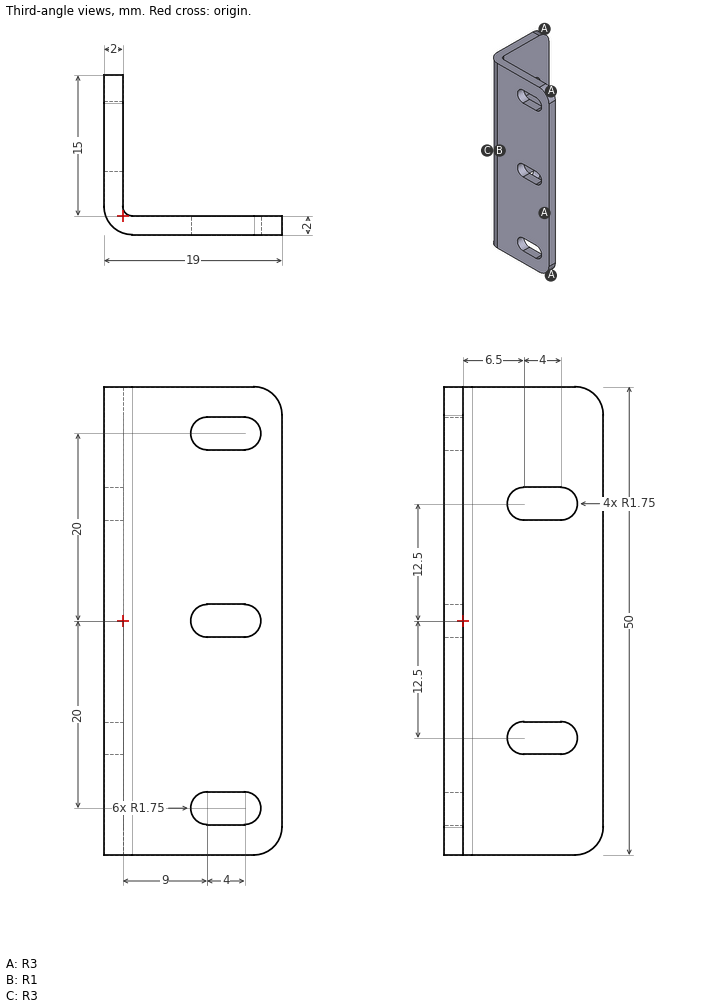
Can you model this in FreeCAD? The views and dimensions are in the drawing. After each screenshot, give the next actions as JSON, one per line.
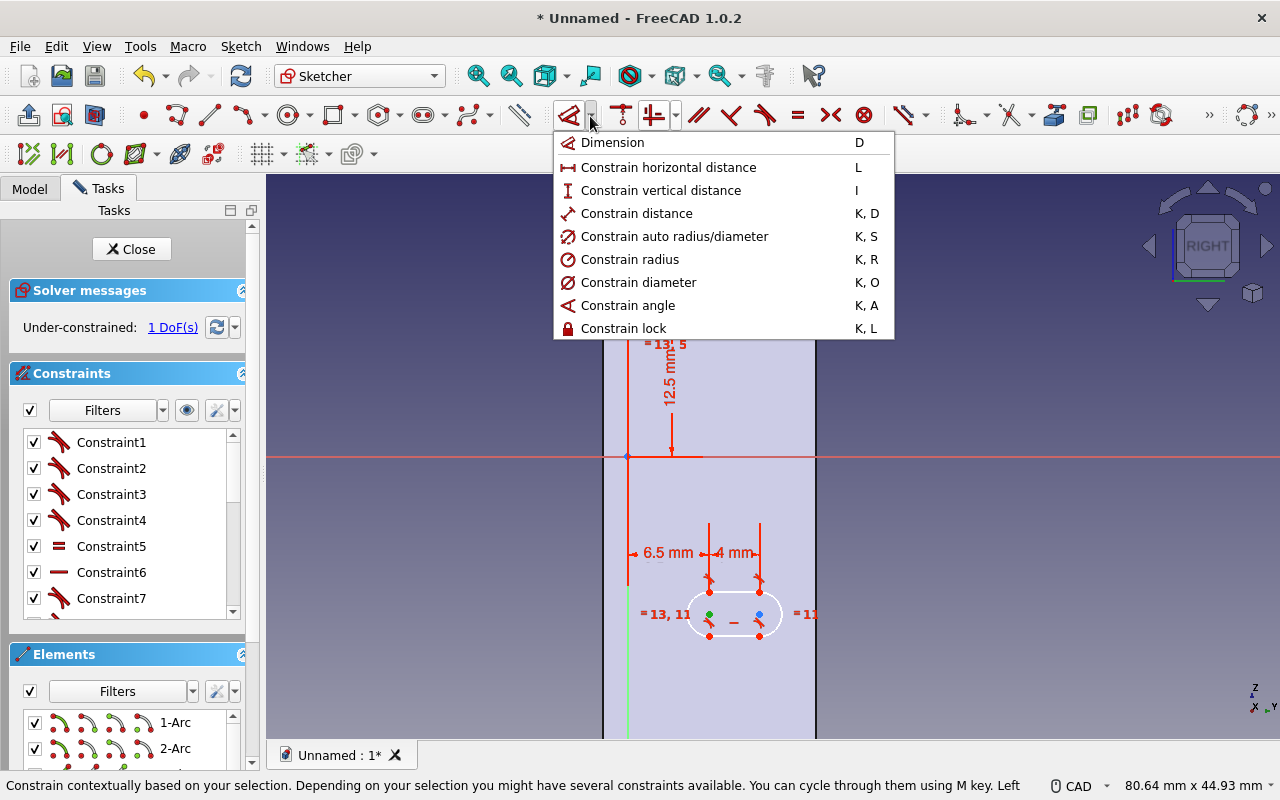
{"action": "left_click", "coordinate": [724, 190]}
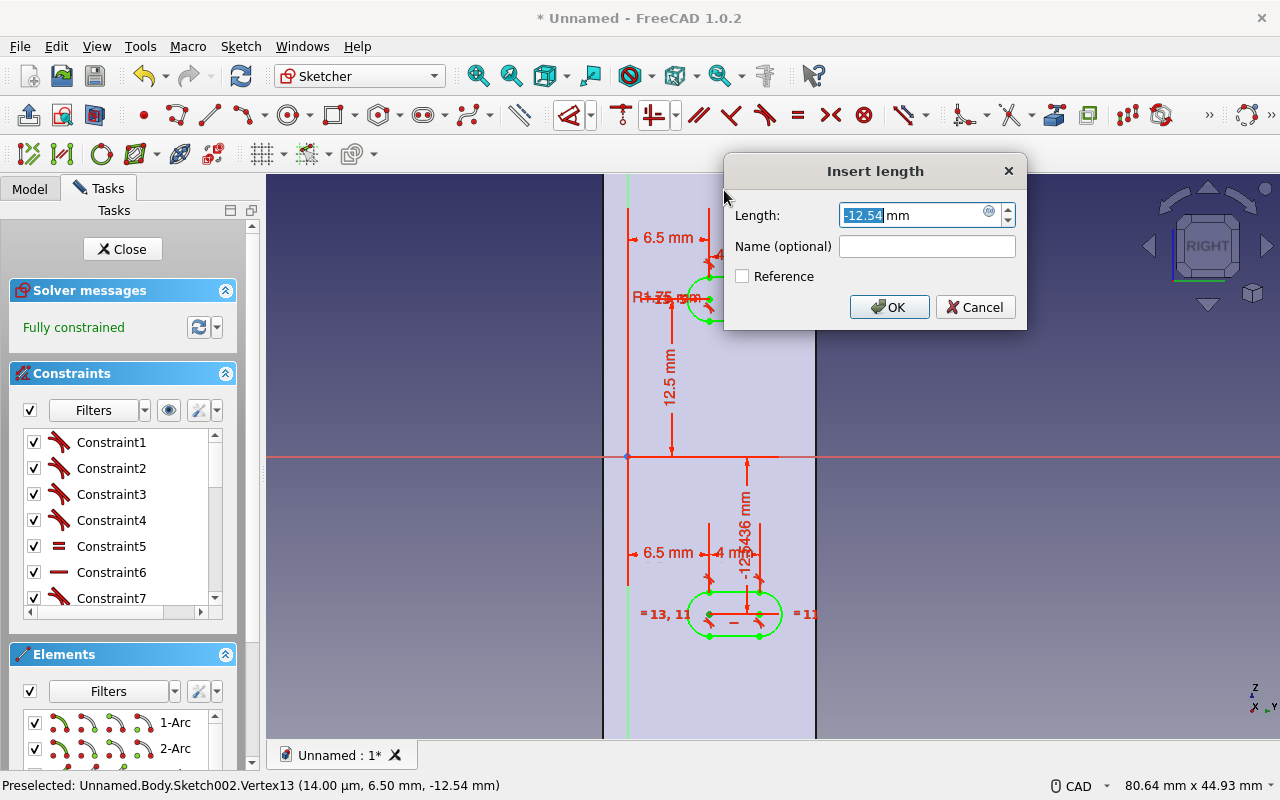
{"action": "type", "text": "-12.5"}
{"action": "key", "text": "Return"}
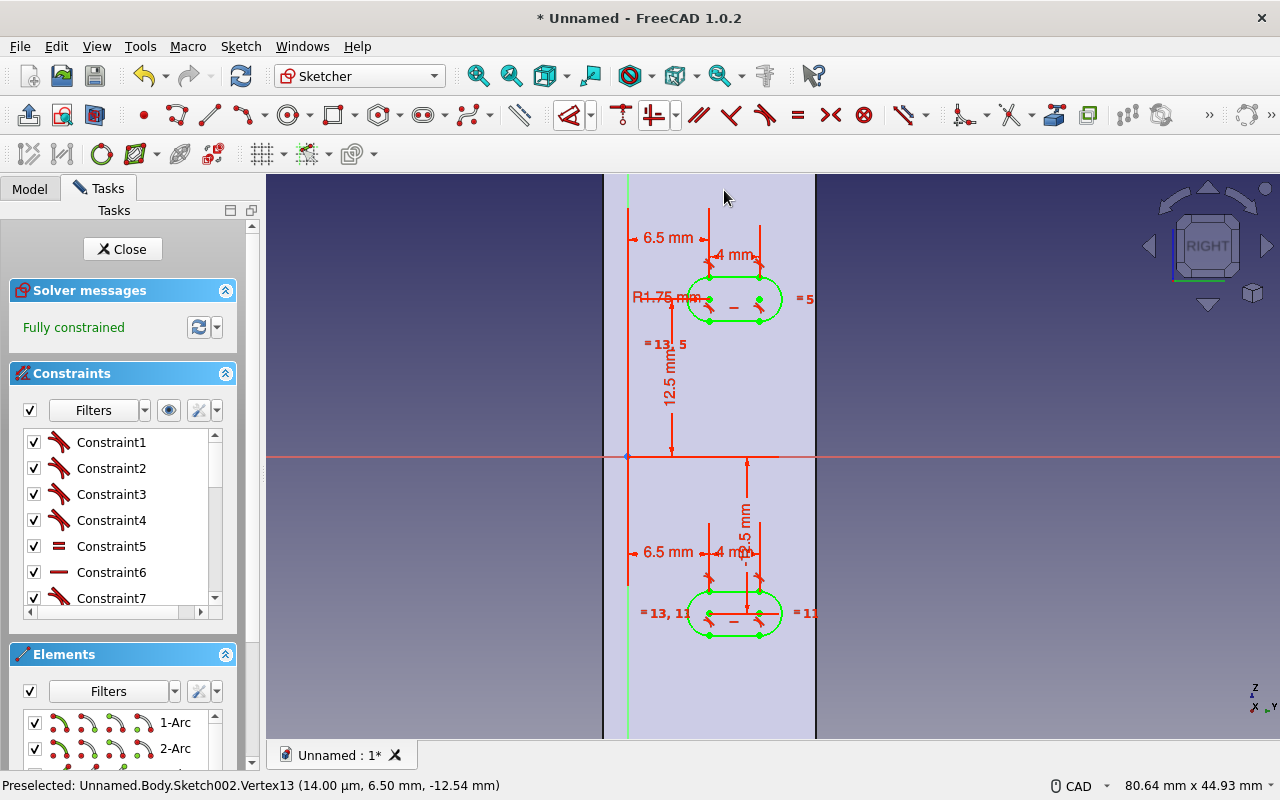
{"action": "left_click", "coordinate": [123, 249]}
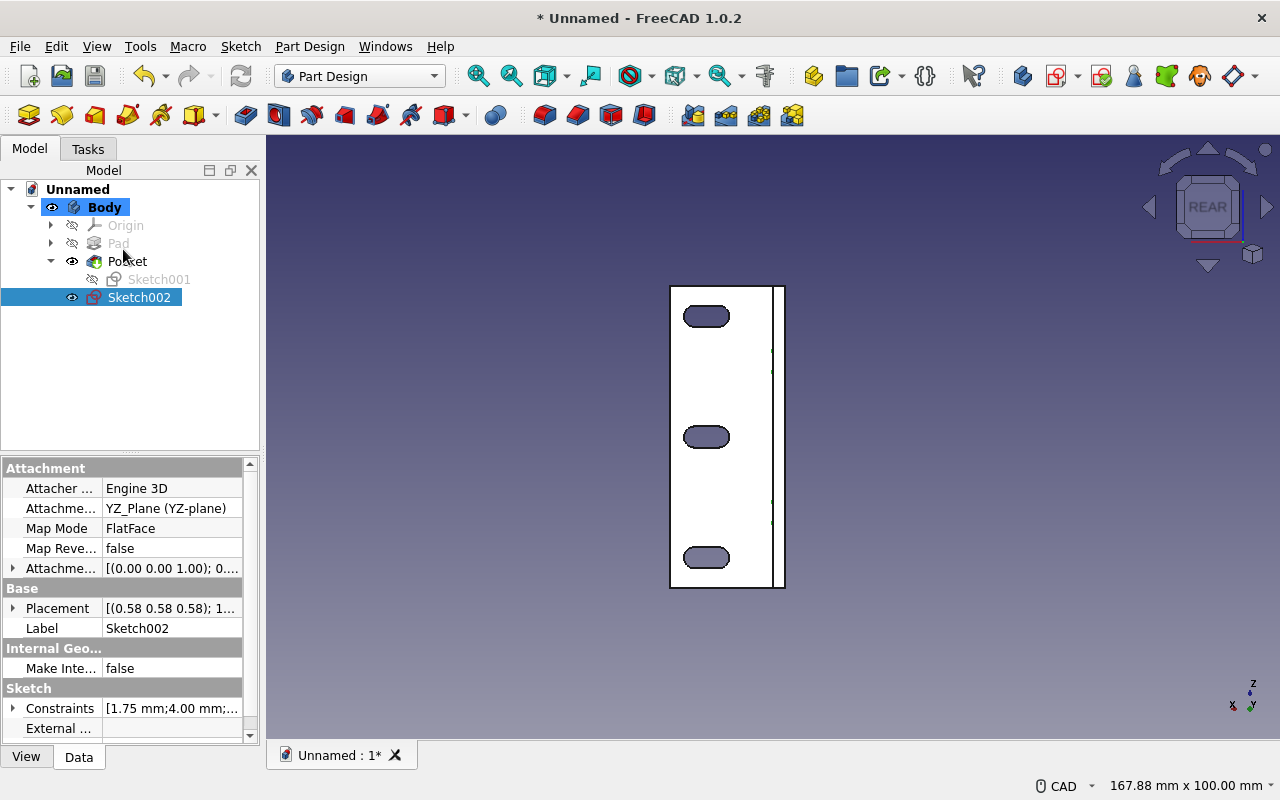
{"action": "left_click", "coordinate": [246, 116]}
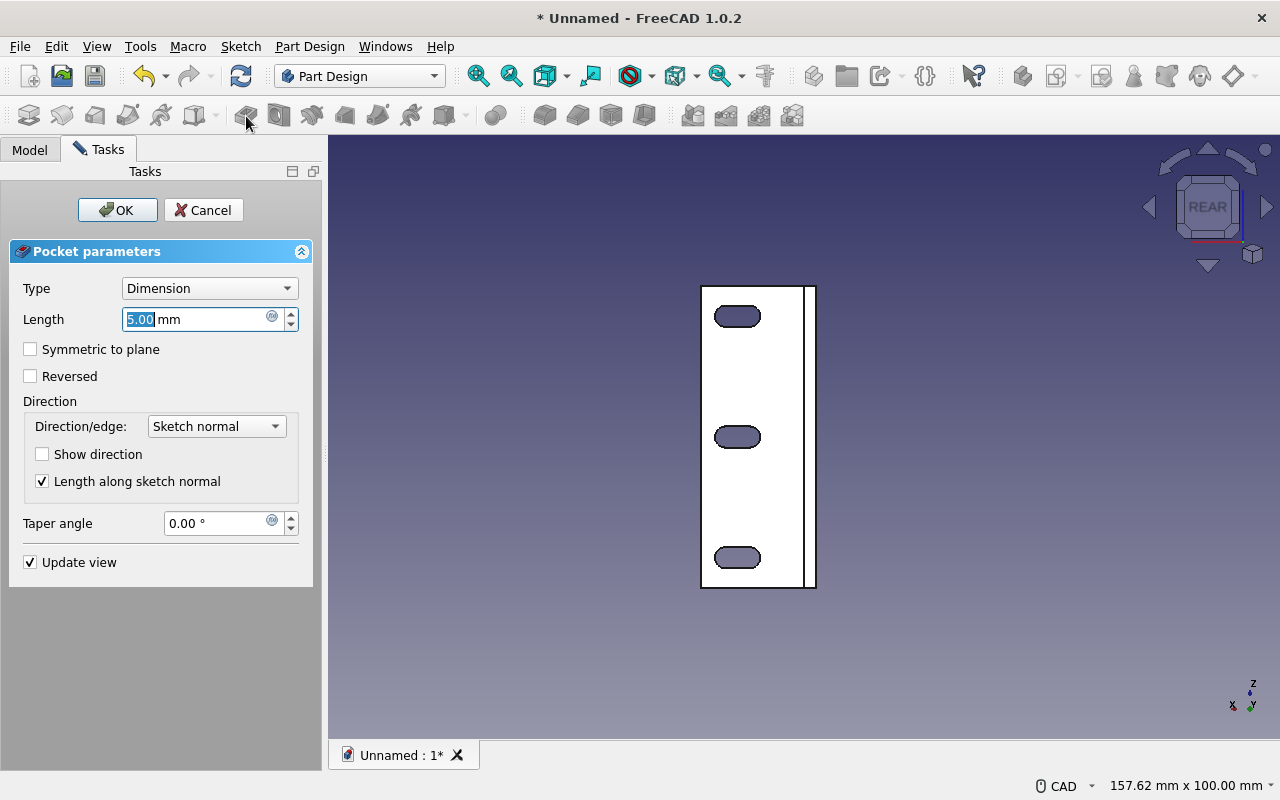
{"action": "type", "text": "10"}
{"action": "key", "text": "Tab"}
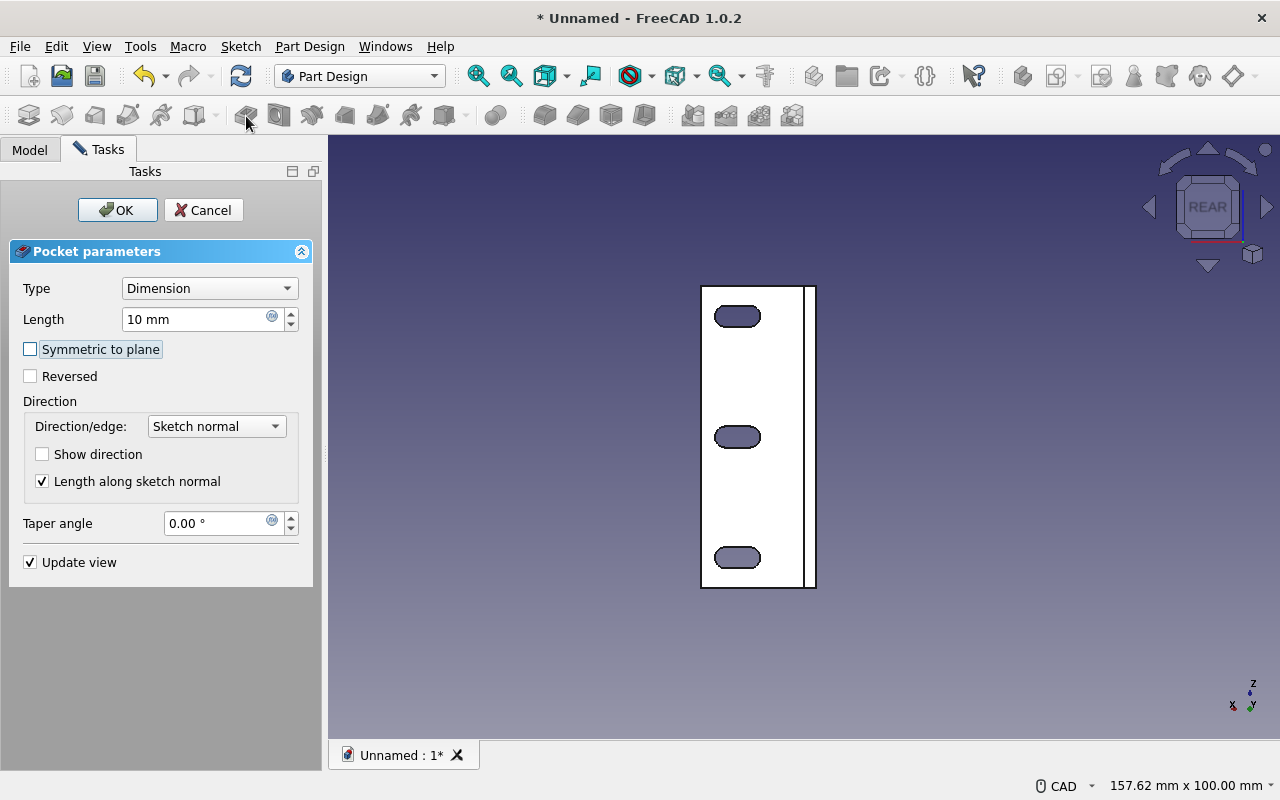
{"action": "left_click", "coordinate": [118, 210]}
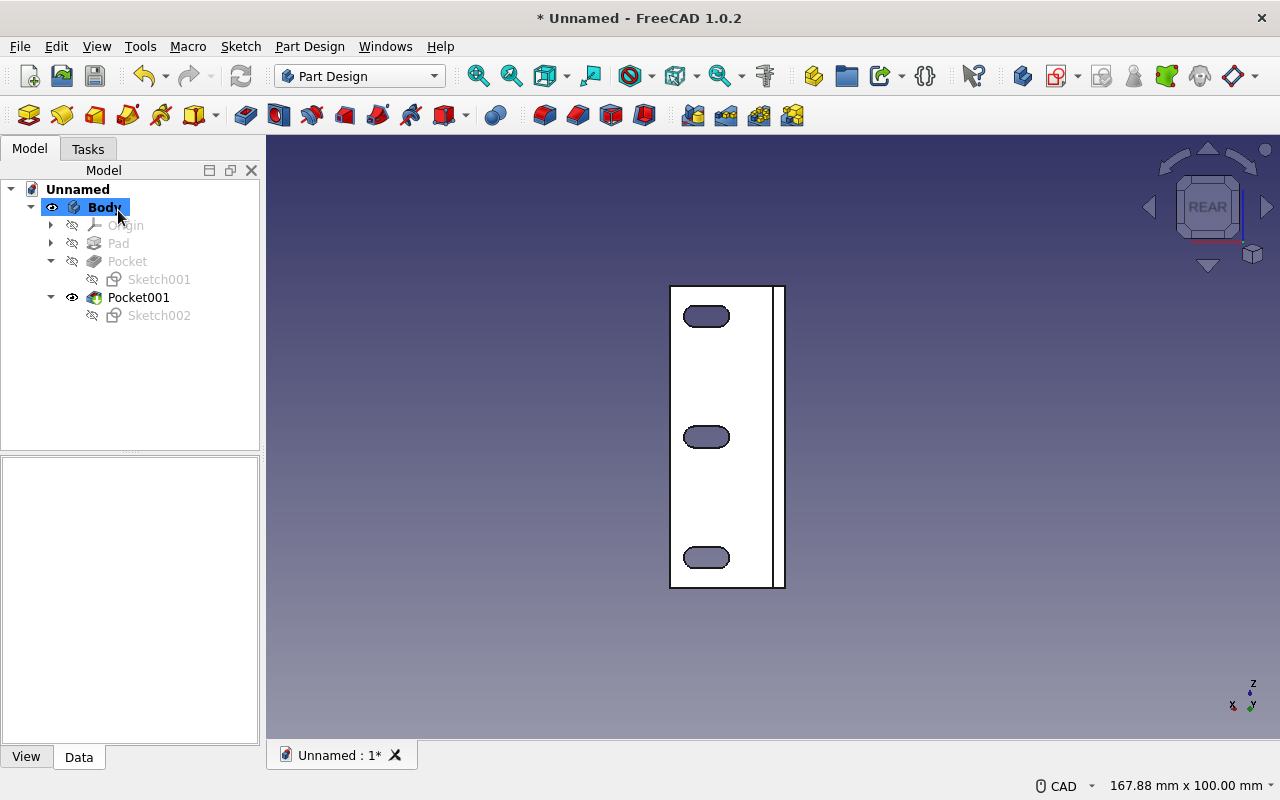
{"action": "left_click", "coordinate": [779, 285]}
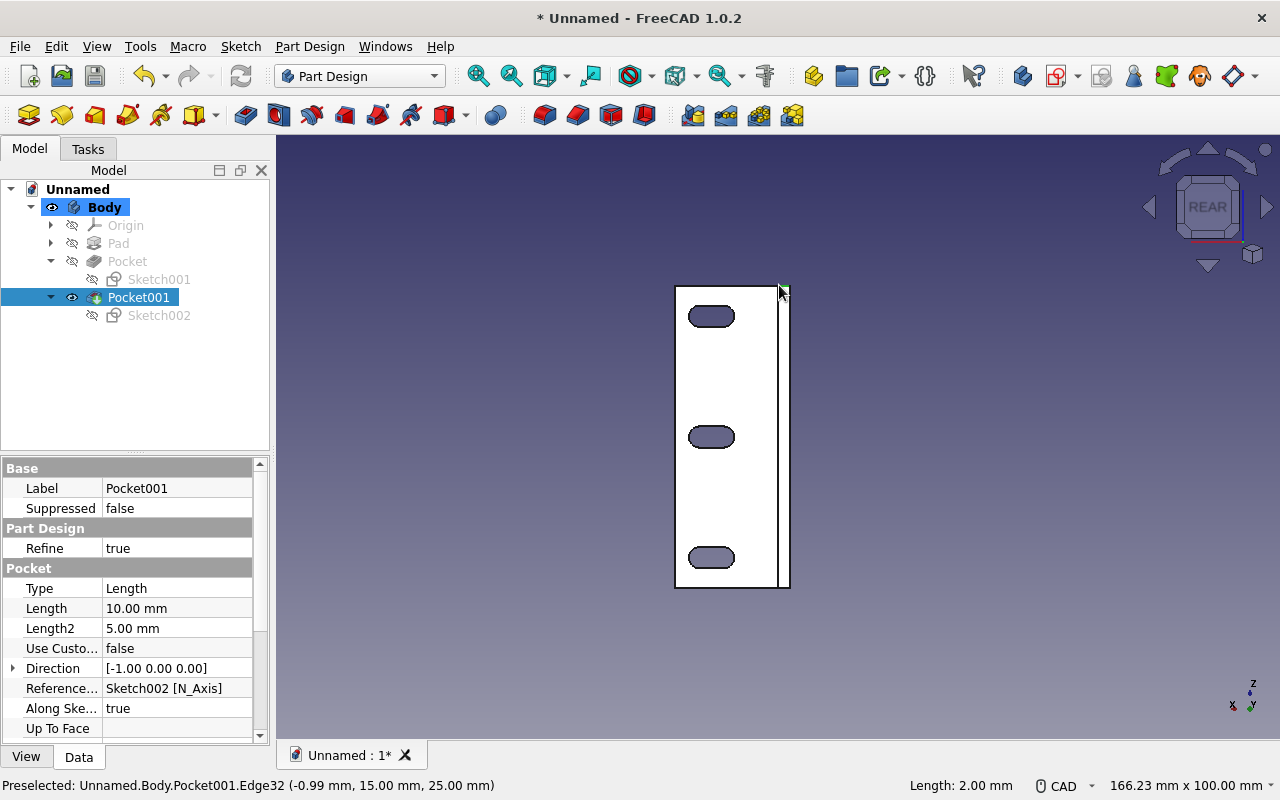
{"action": "scroll", "coordinate": [784, 587], "scroll_direction": "up", "scroll_amount": 6}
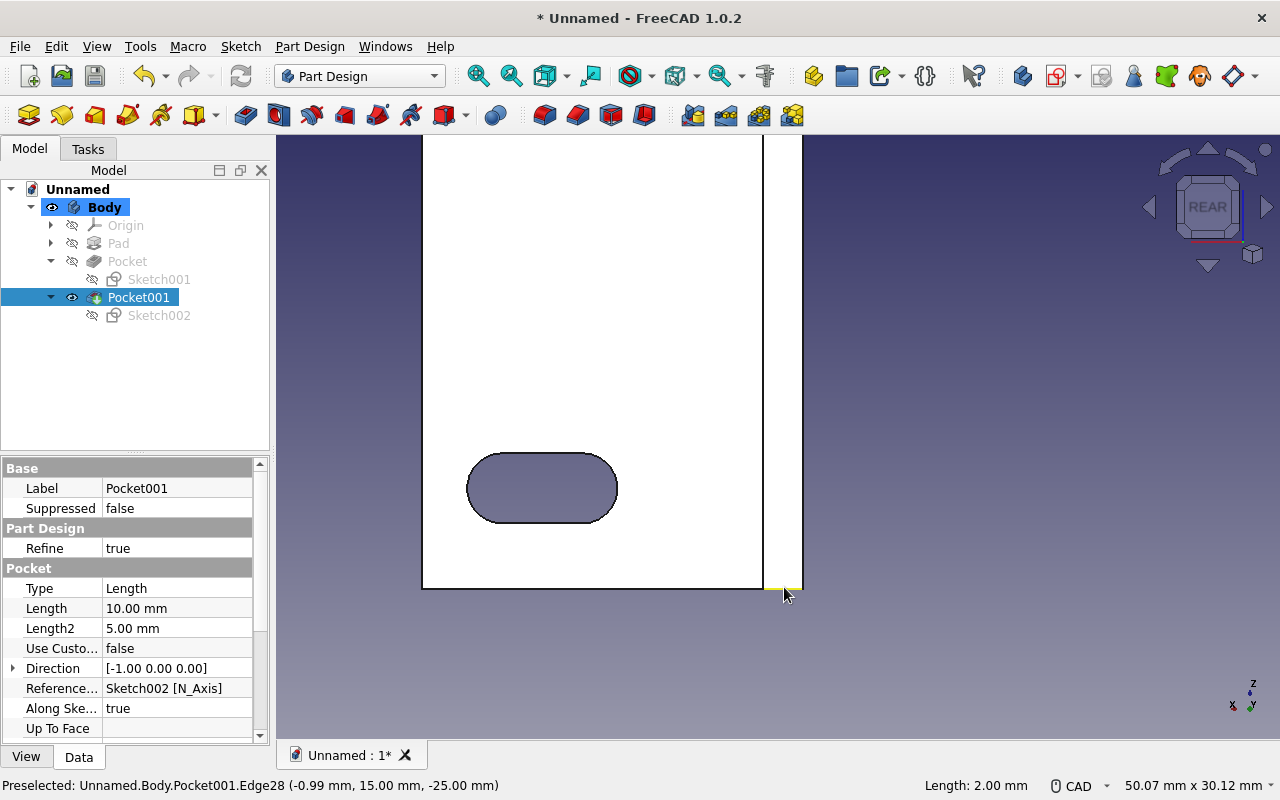
{"action": "left_click", "coordinate": [783, 588], "text": "ctrl"}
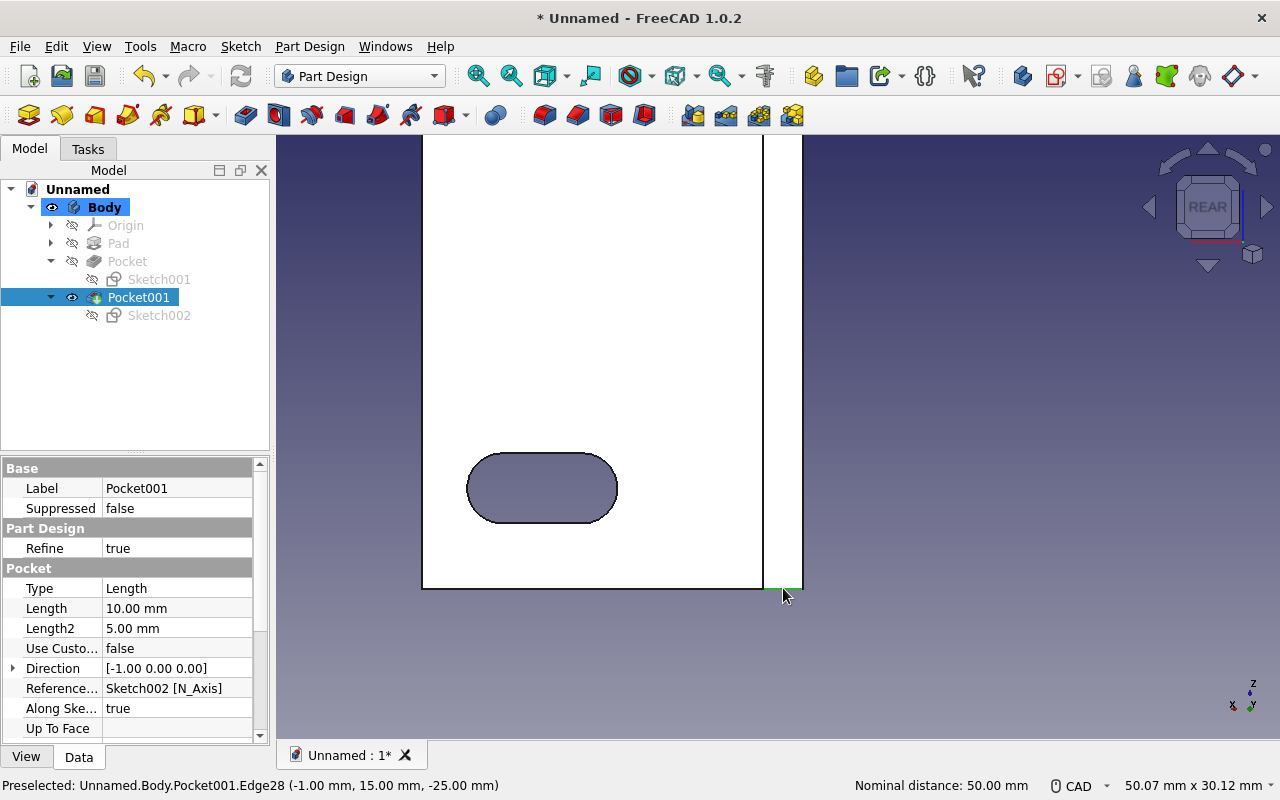
{"action": "left_click", "coordinate": [479, 76]}